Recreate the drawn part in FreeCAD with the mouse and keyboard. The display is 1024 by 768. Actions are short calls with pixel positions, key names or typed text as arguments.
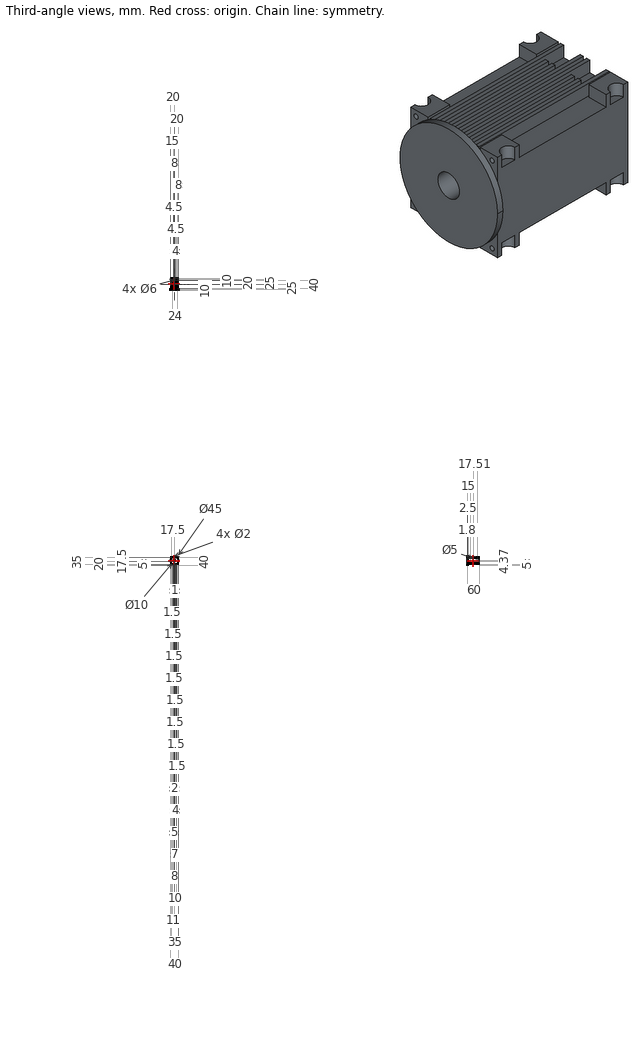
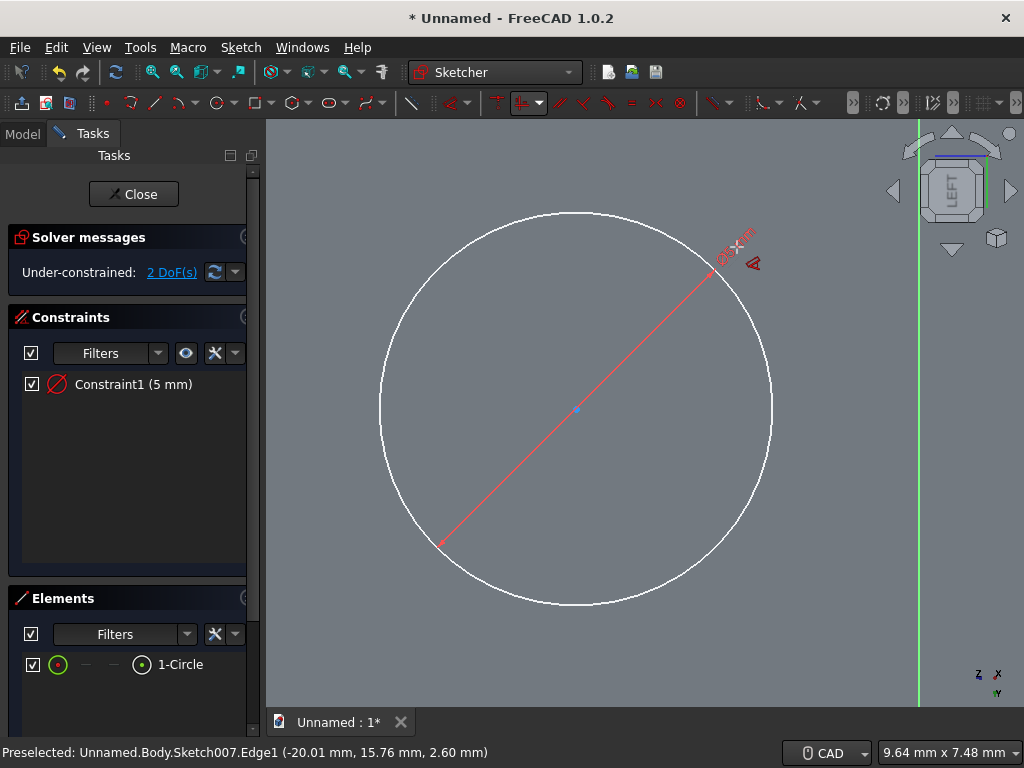
click(576, 409)
click(717, 443)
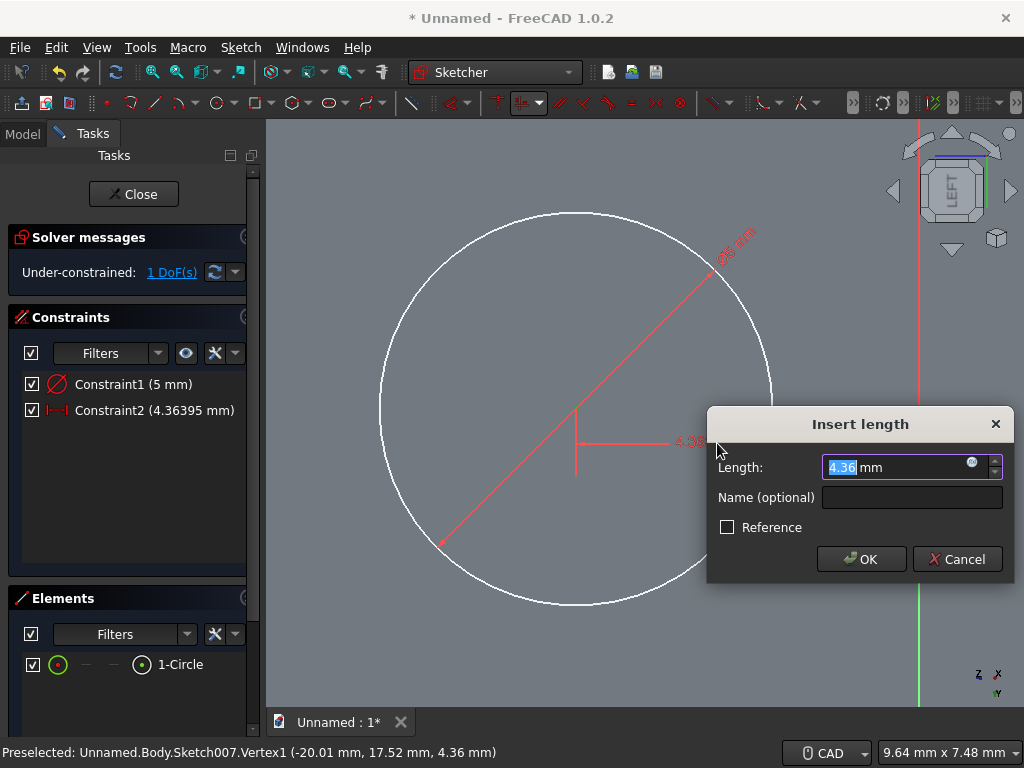
text(4.37)
key(Return)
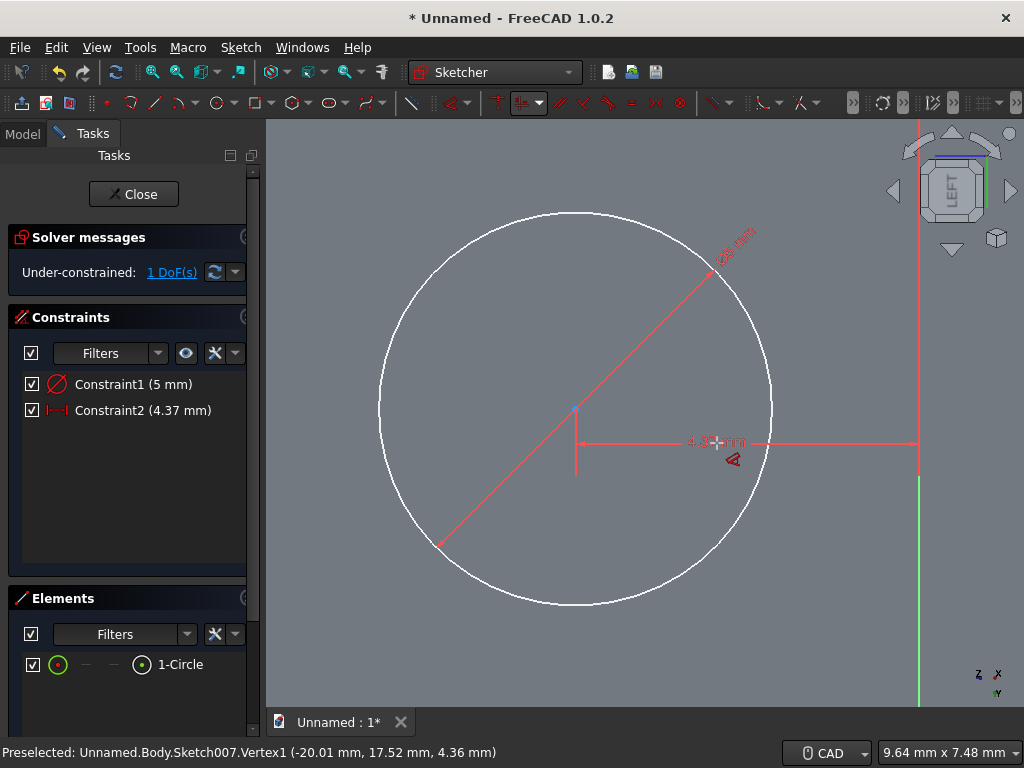
click(576, 409)
click(542, 278)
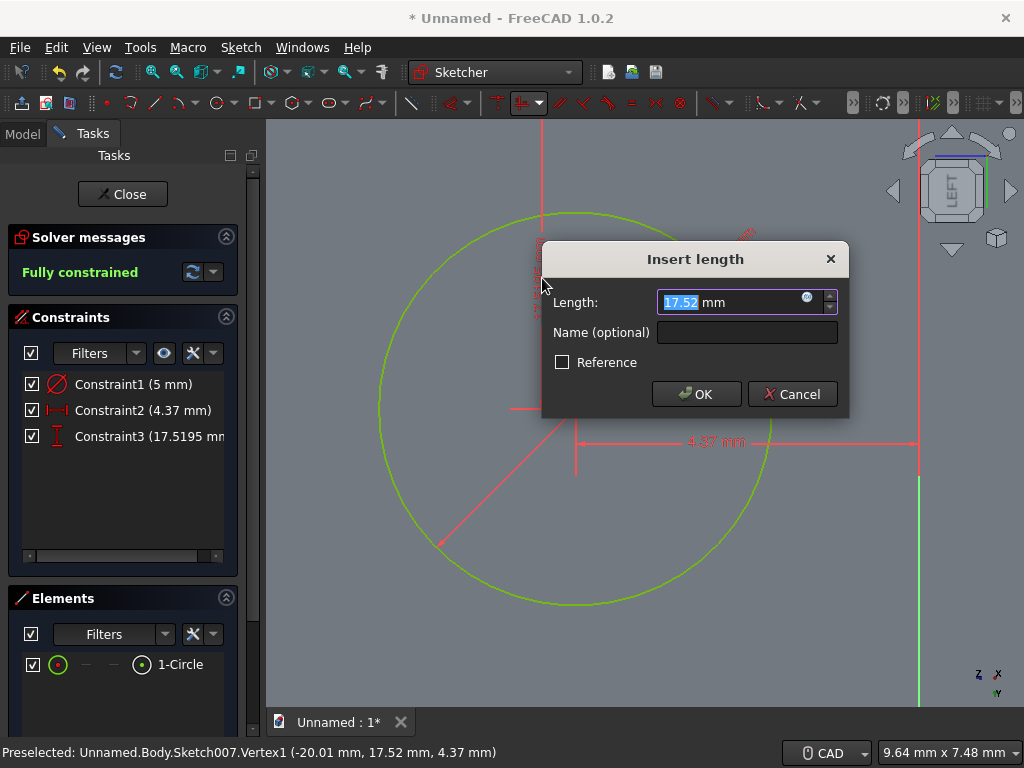
text(17.51)
key(Return)
key(Escape)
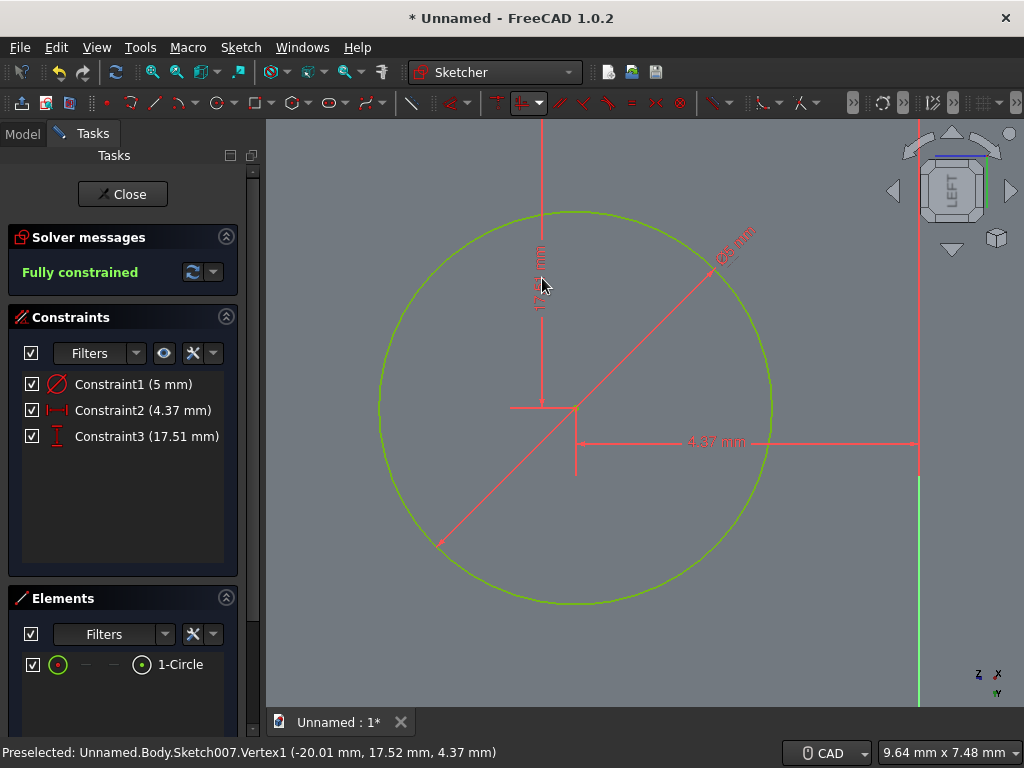
click(123, 194)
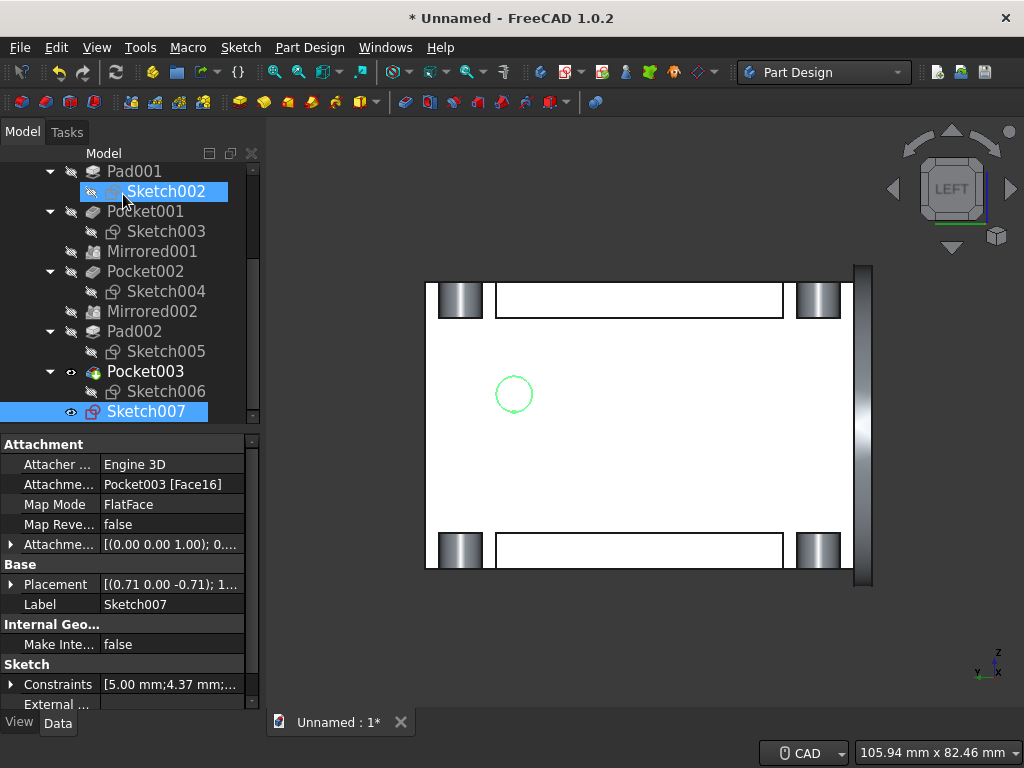
click(406, 102)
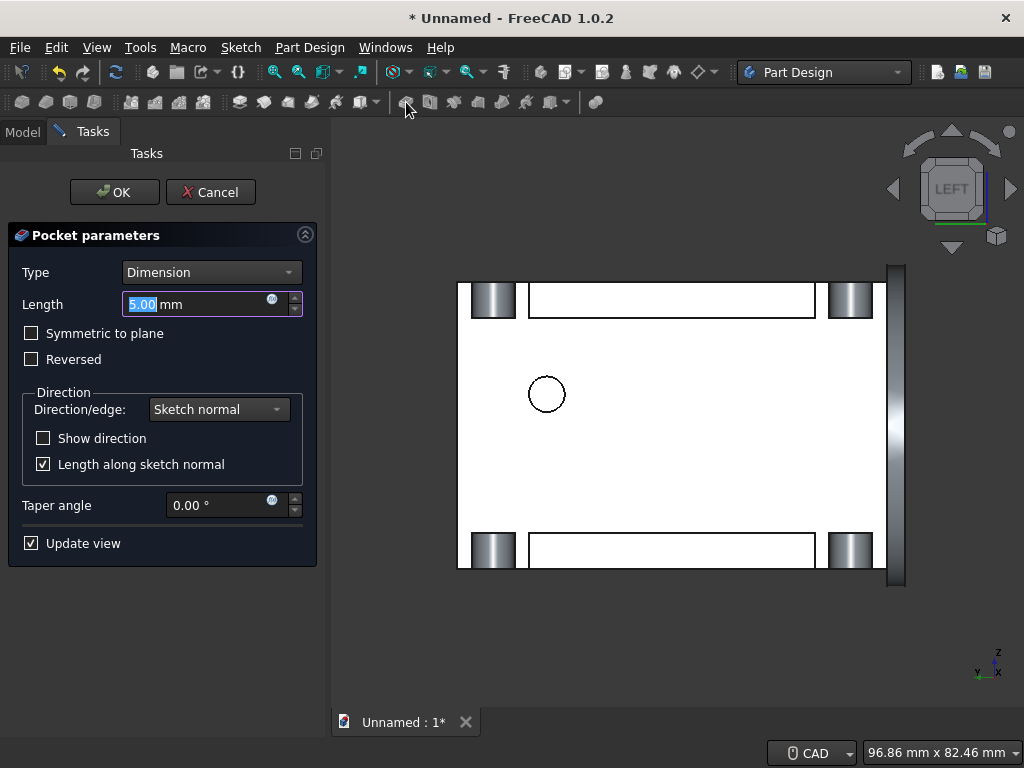
text(15)
key(Tab)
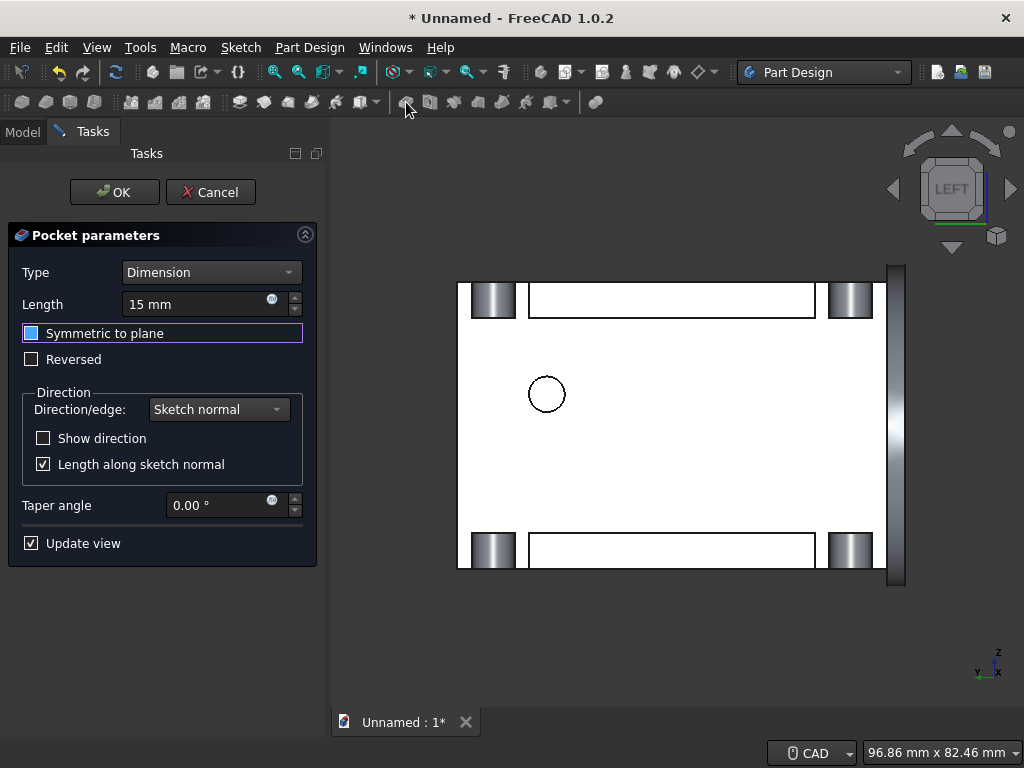
click(115, 192)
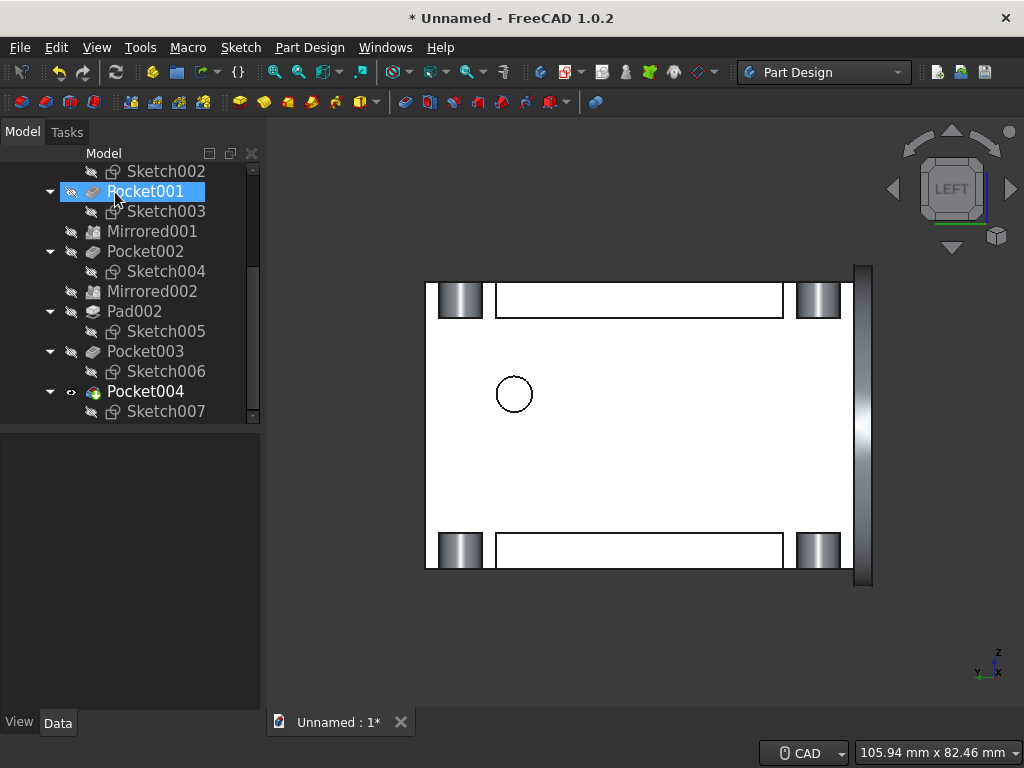
key(4)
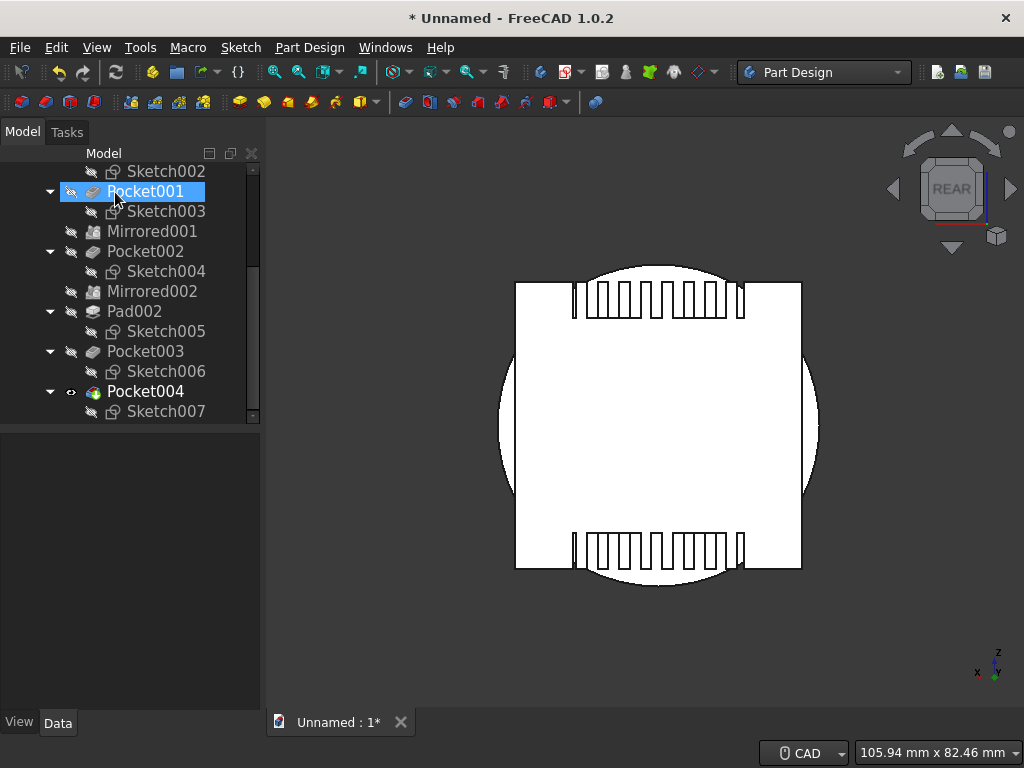
key(5)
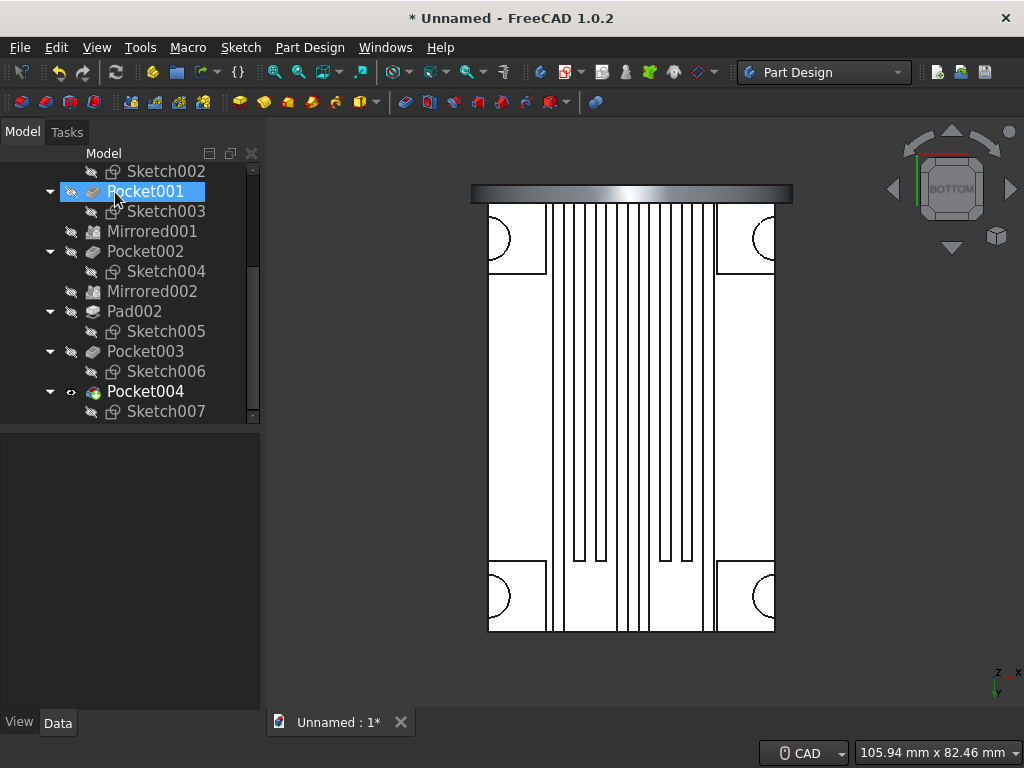
key(3)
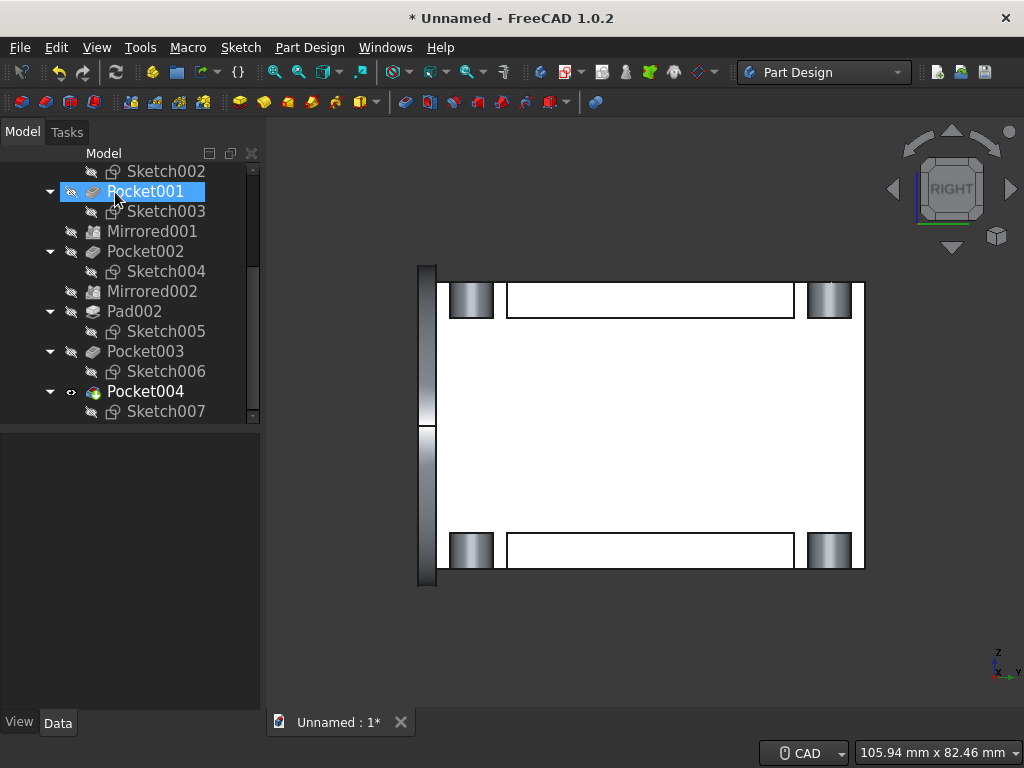
scroll(160, 287, down, 3)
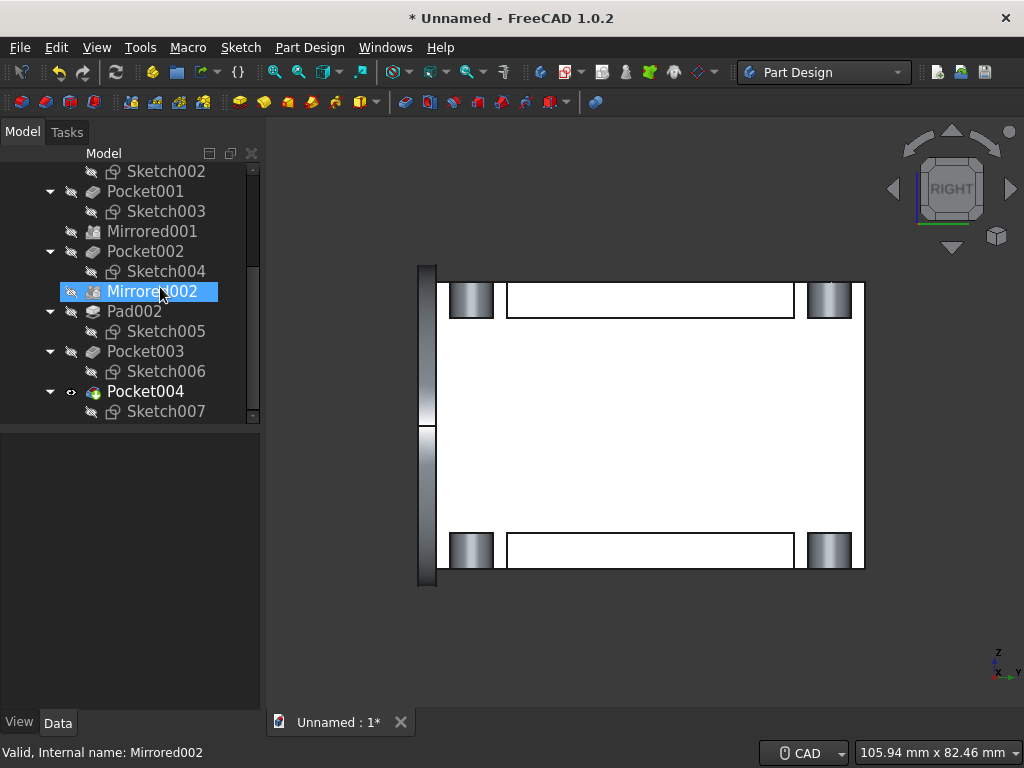
scroll(160, 287, up, 15)